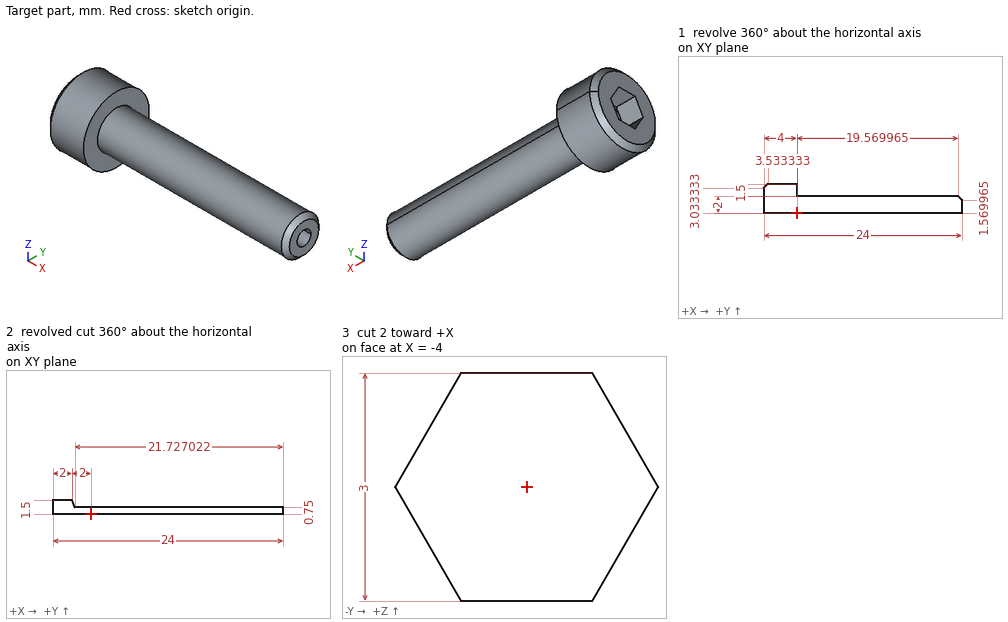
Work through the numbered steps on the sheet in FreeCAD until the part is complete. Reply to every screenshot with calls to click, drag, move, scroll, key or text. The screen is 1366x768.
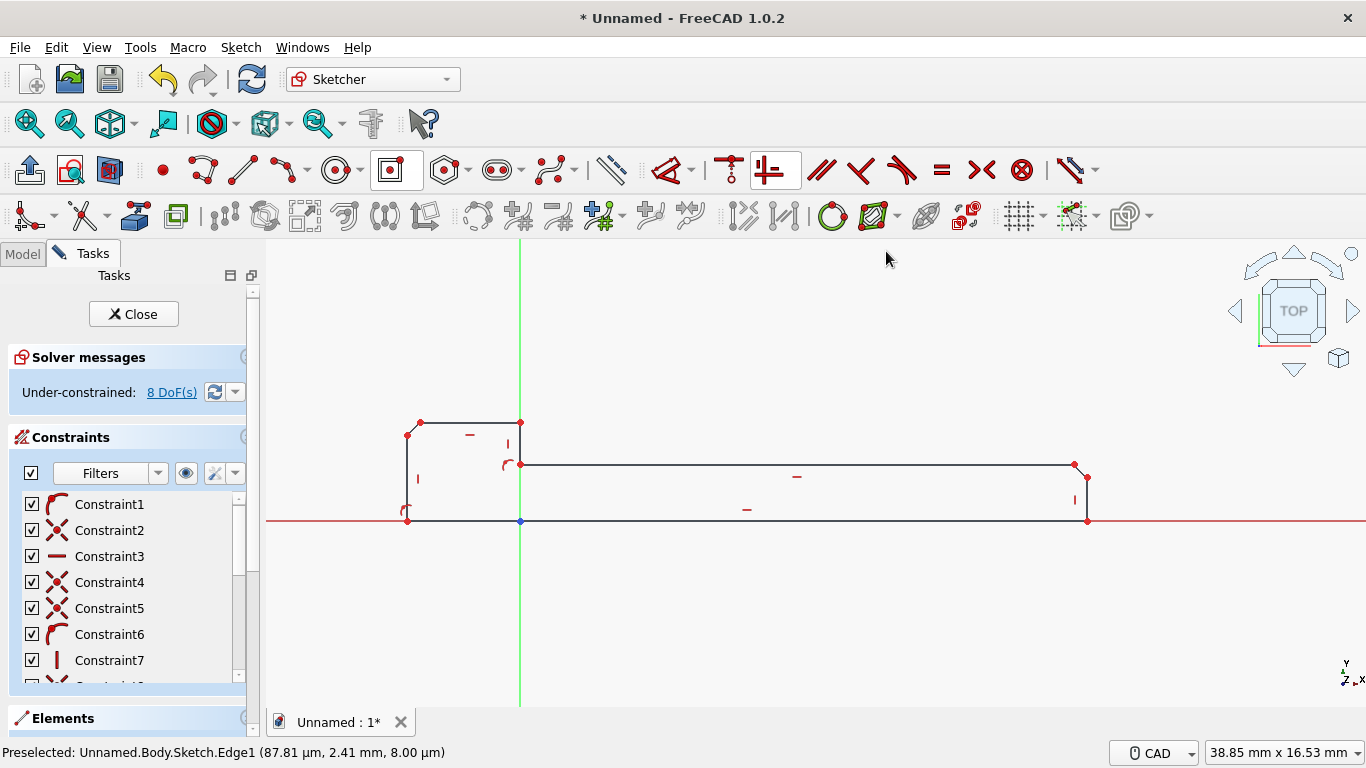
key(d)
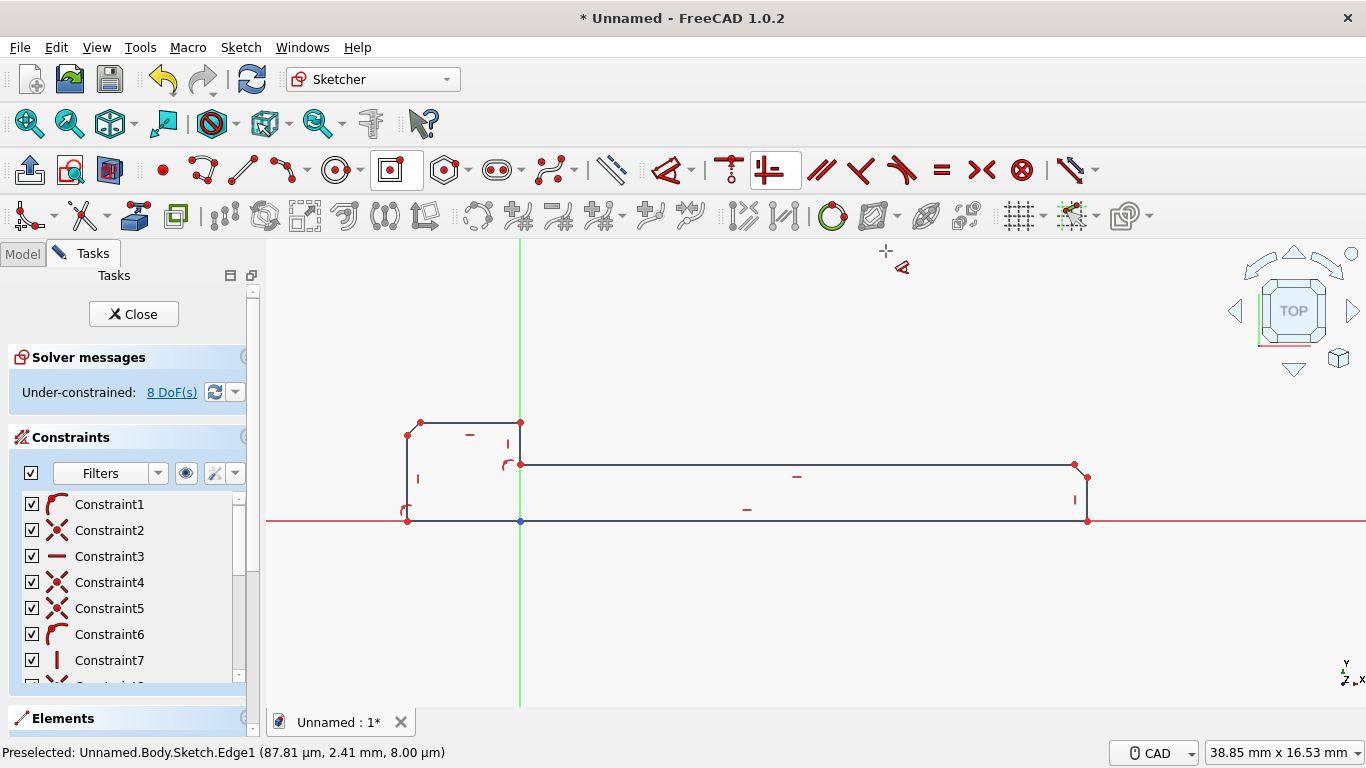
click(611, 521)
click(747, 555)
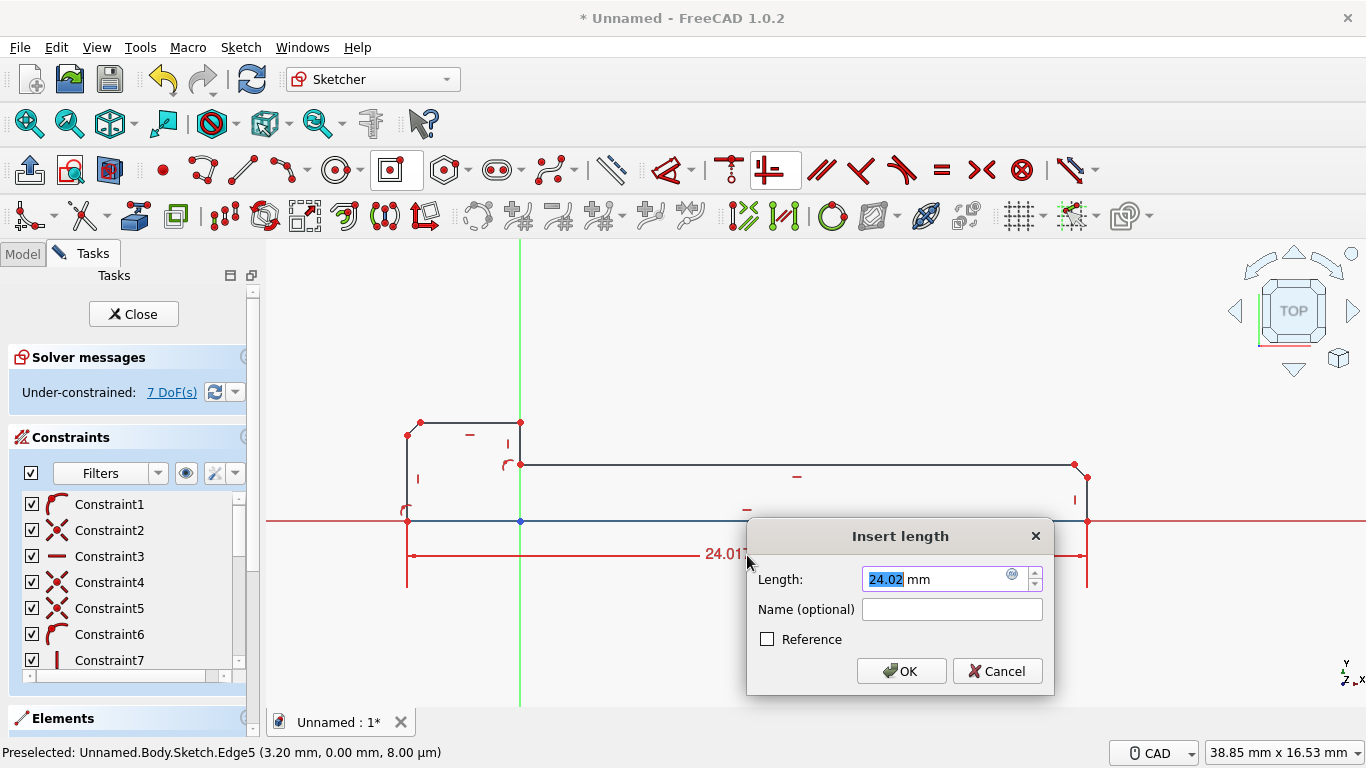
text(24)
key(Return)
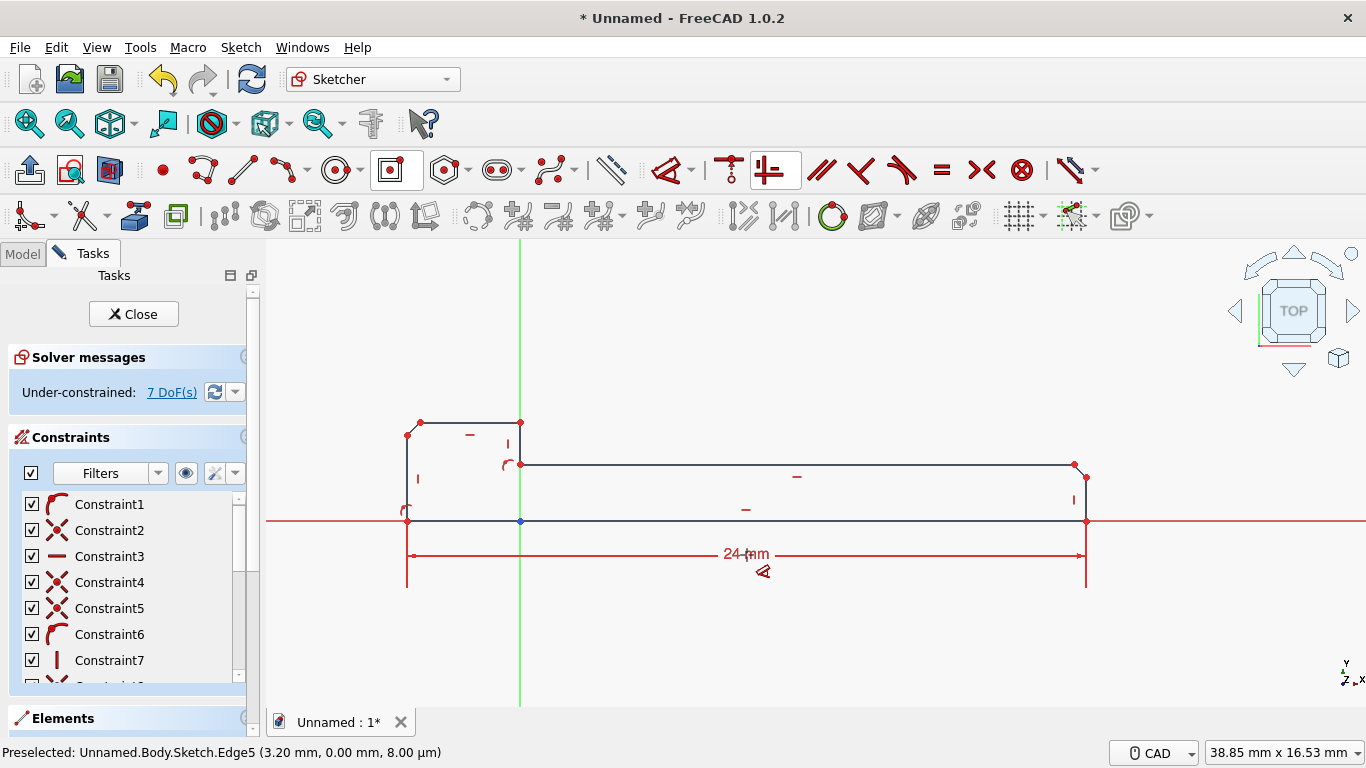
click(520, 465)
click(486, 493)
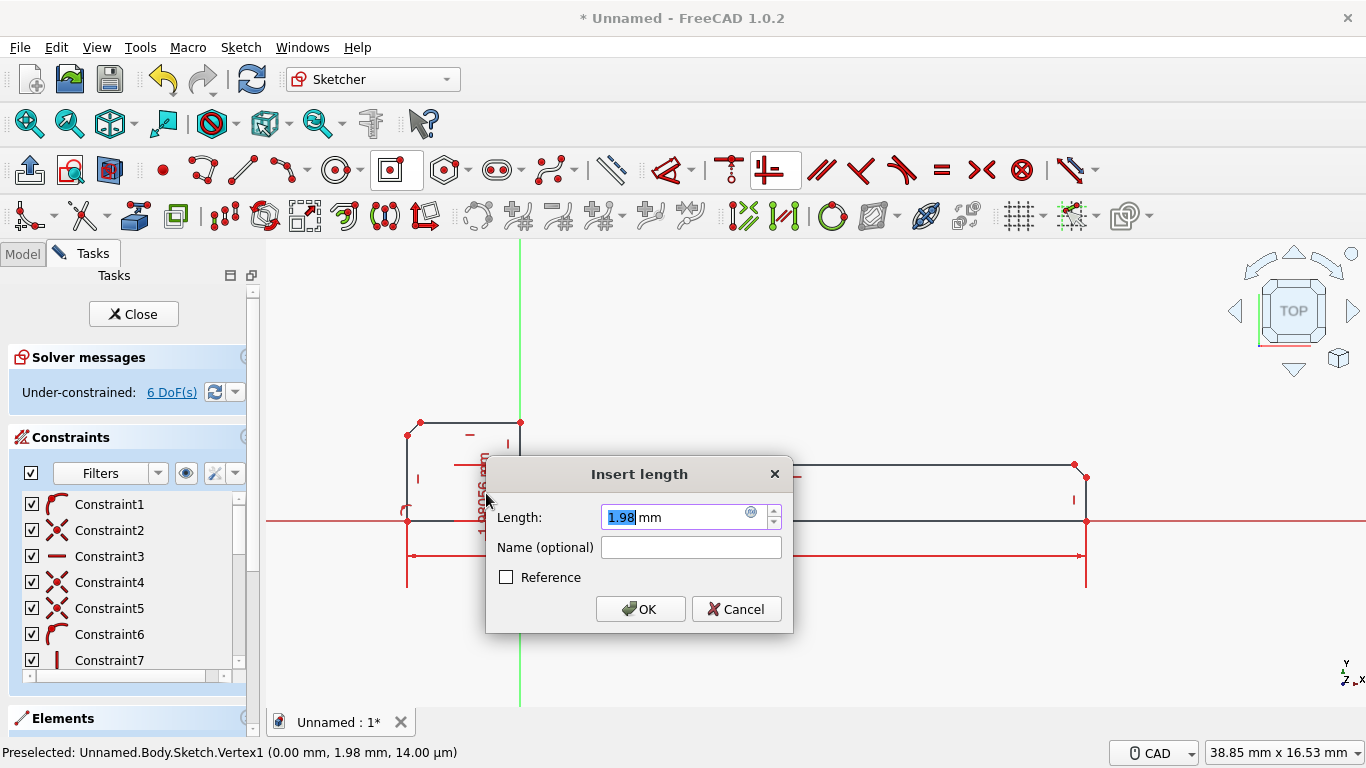
text(2)
key(Return)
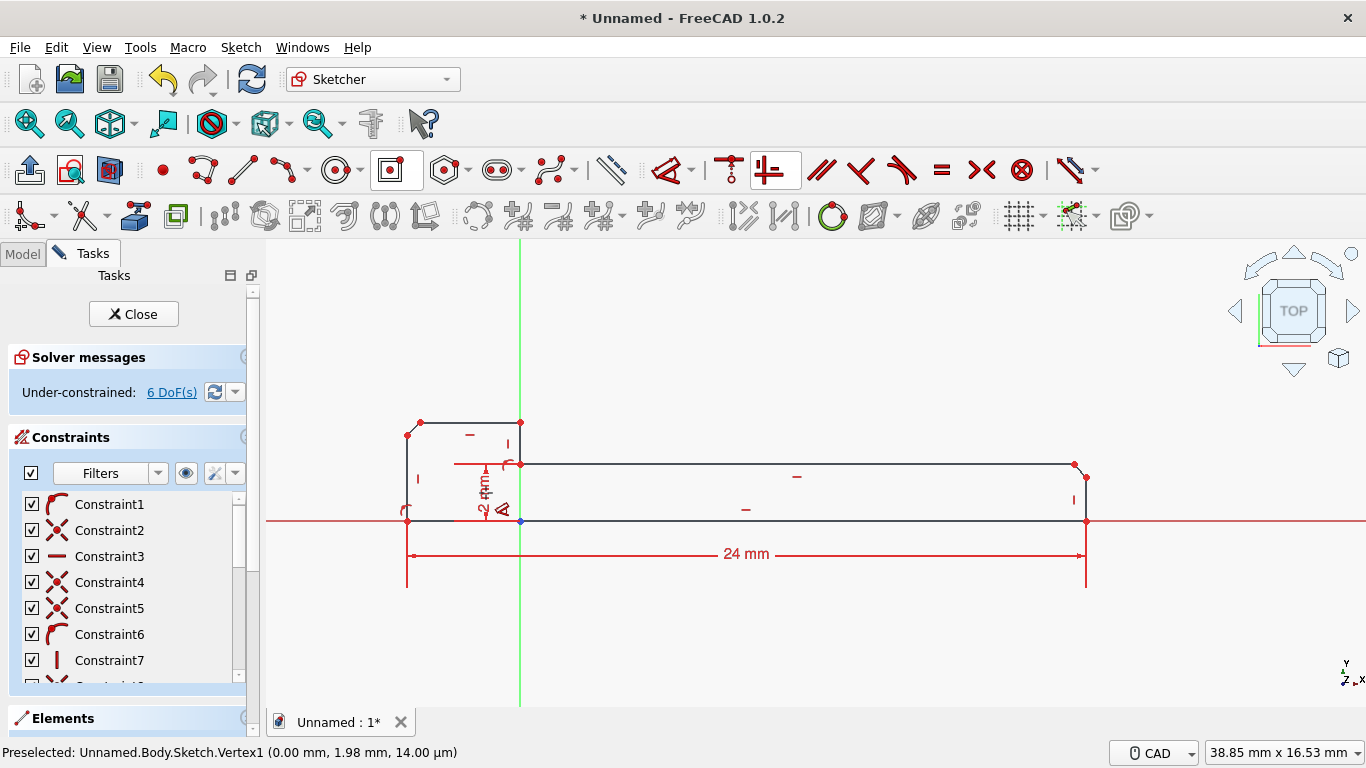
click(407, 436)
click(464, 555)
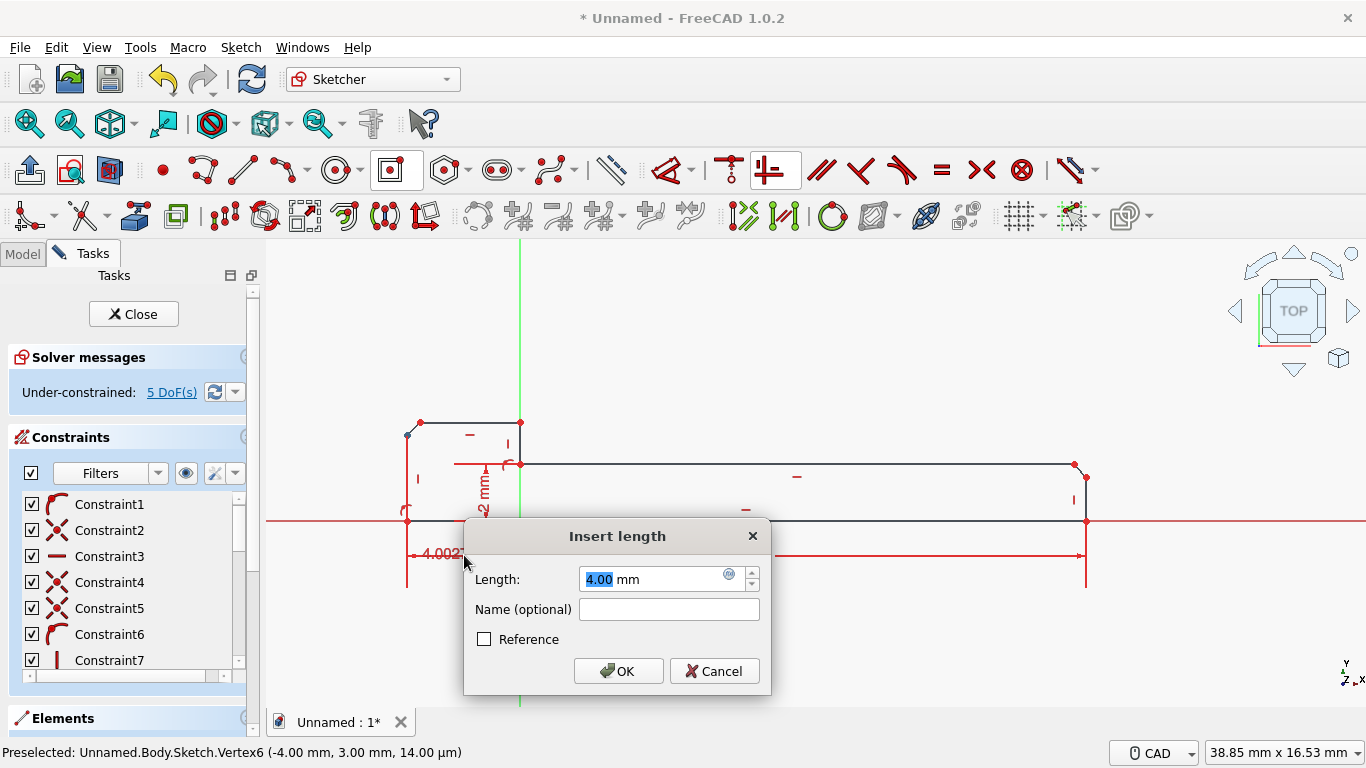
text(4)
key(Return)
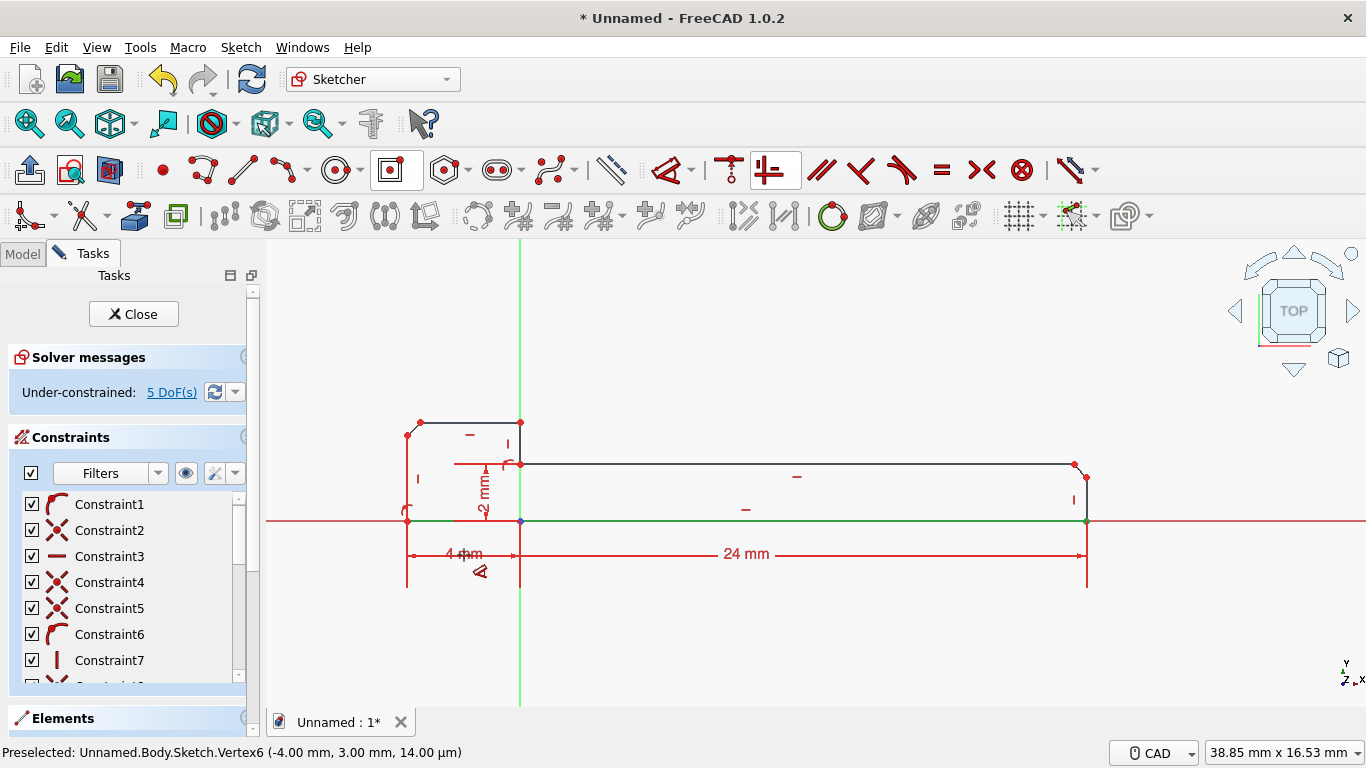
click(520, 452)
click(486, 444)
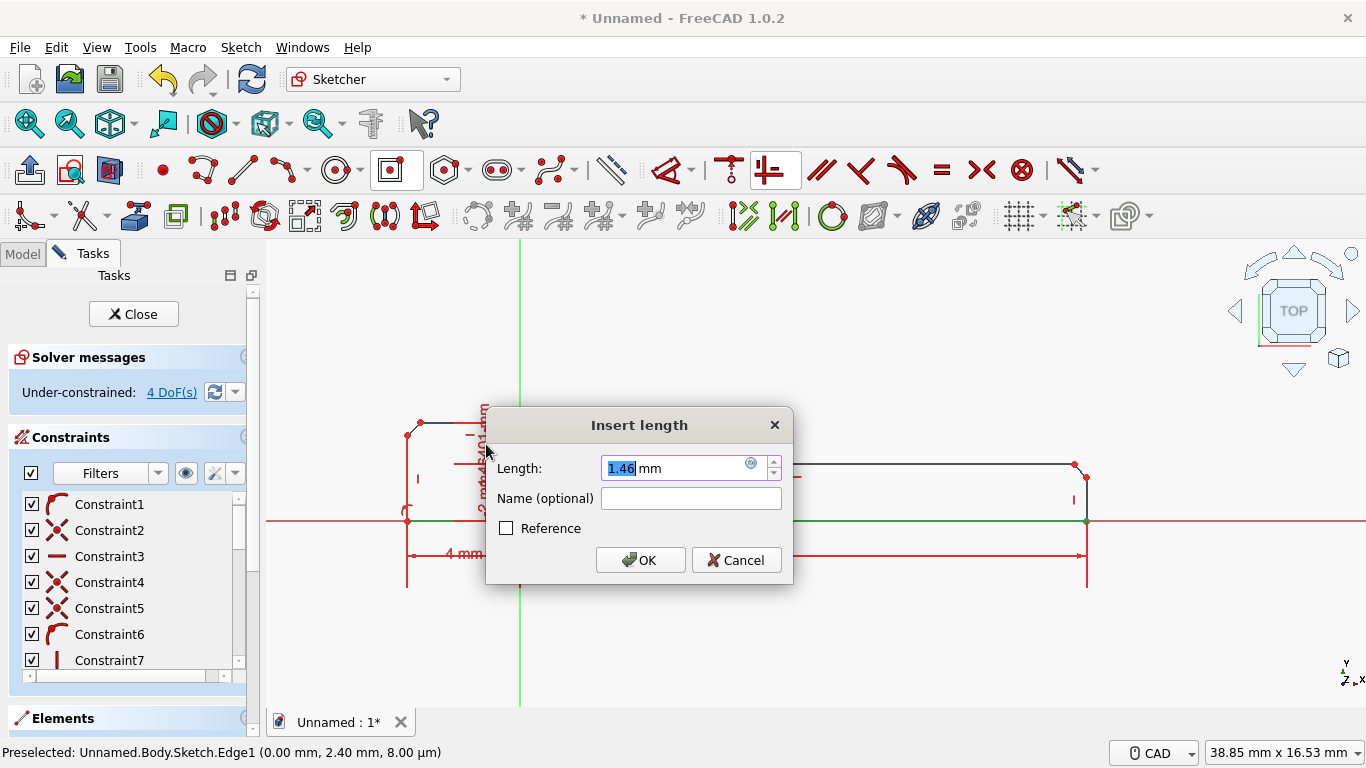
text(1.5)
key(Return)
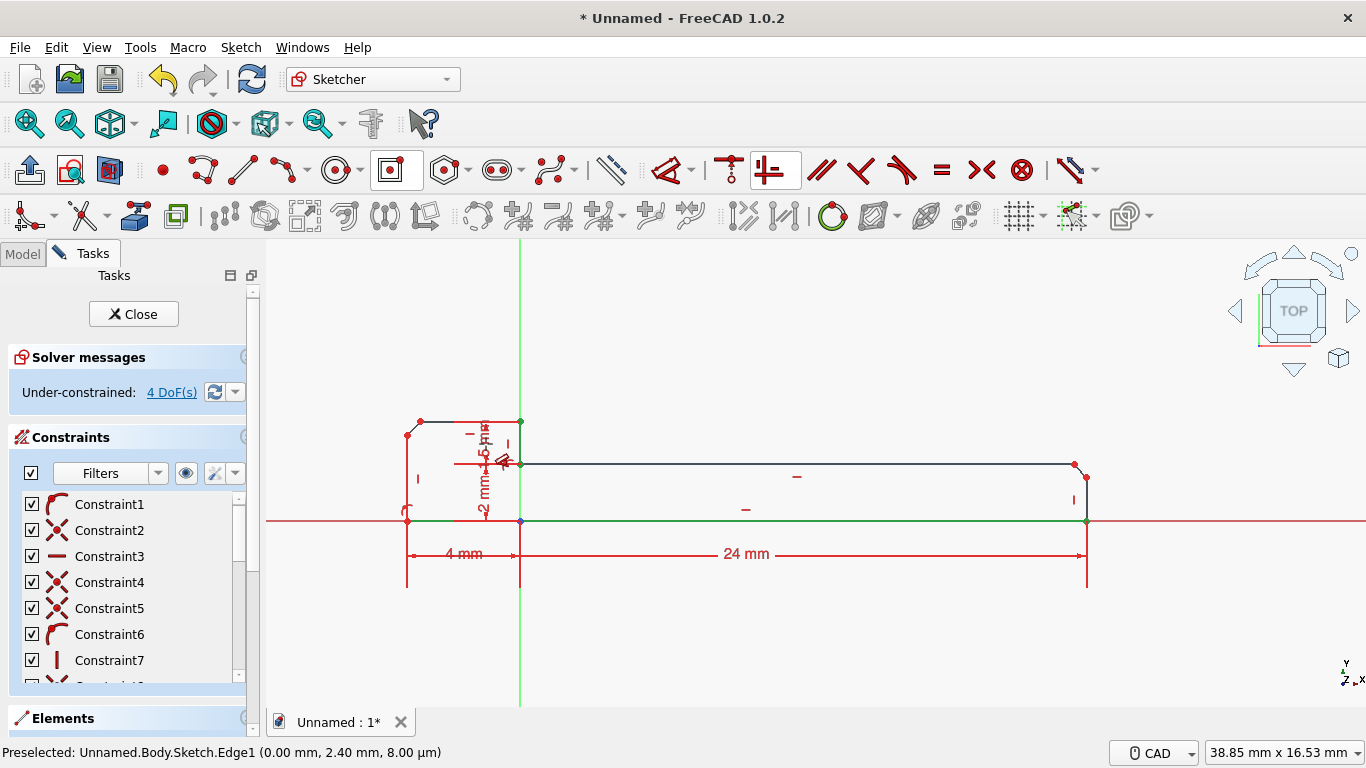
click(490, 422)
click(470, 388)